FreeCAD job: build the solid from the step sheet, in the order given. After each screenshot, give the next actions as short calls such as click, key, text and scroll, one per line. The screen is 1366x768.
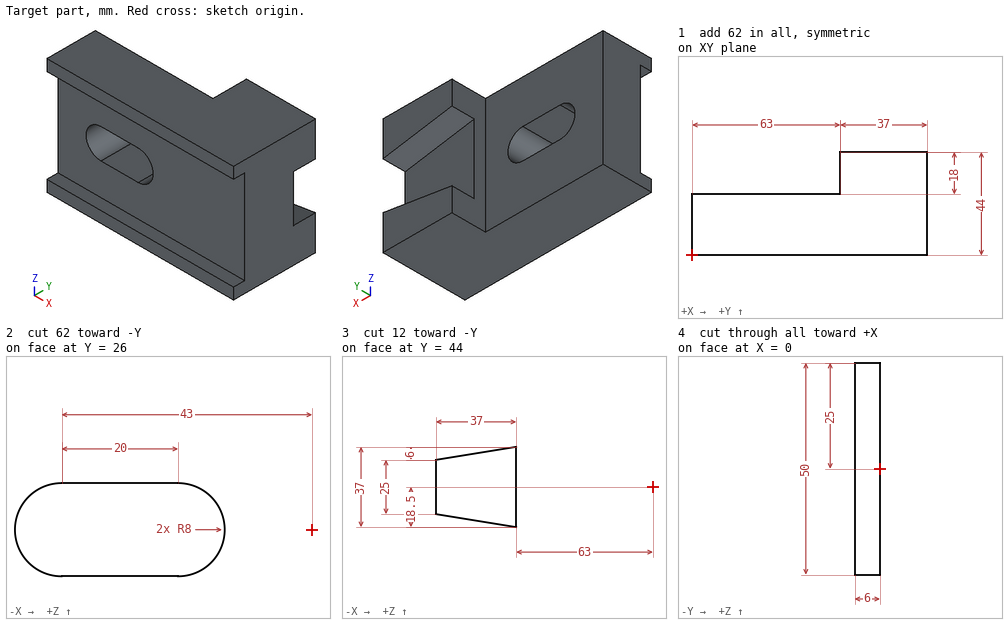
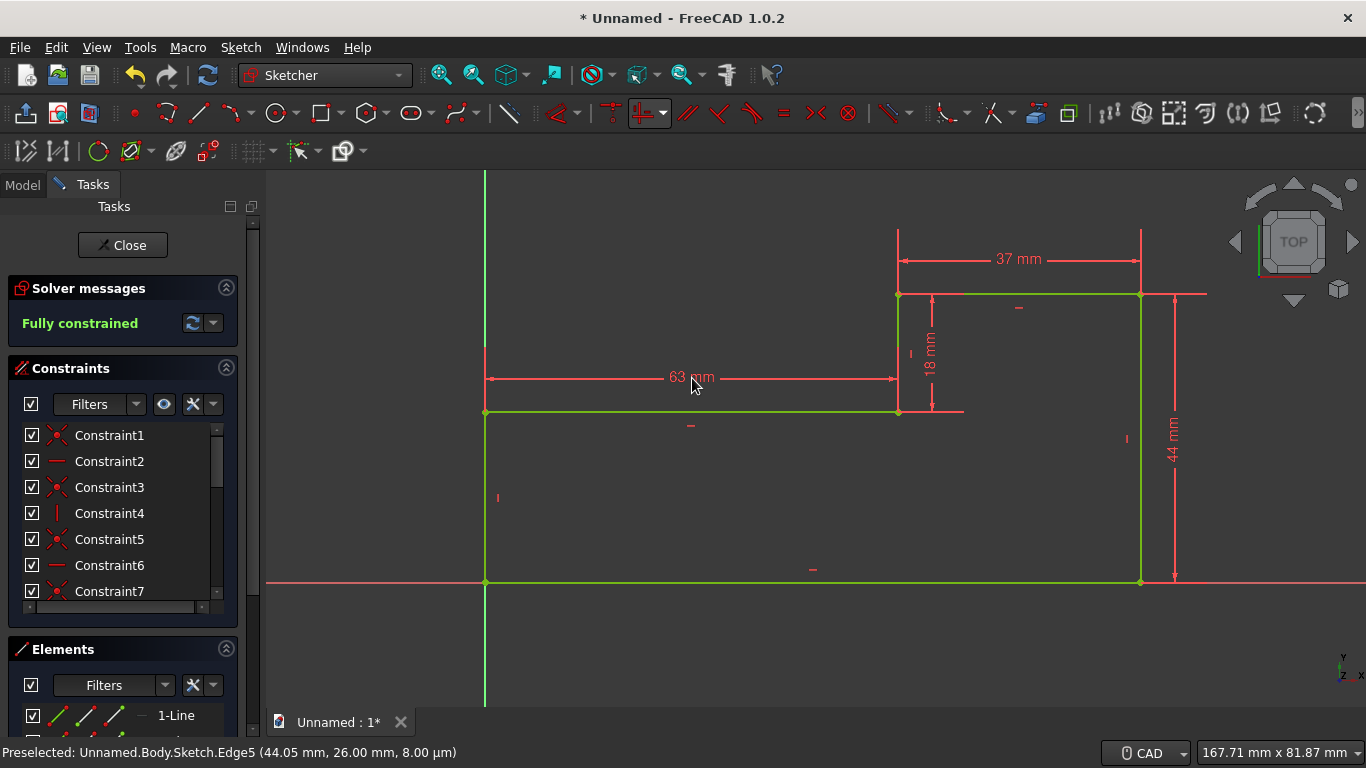
click(123, 245)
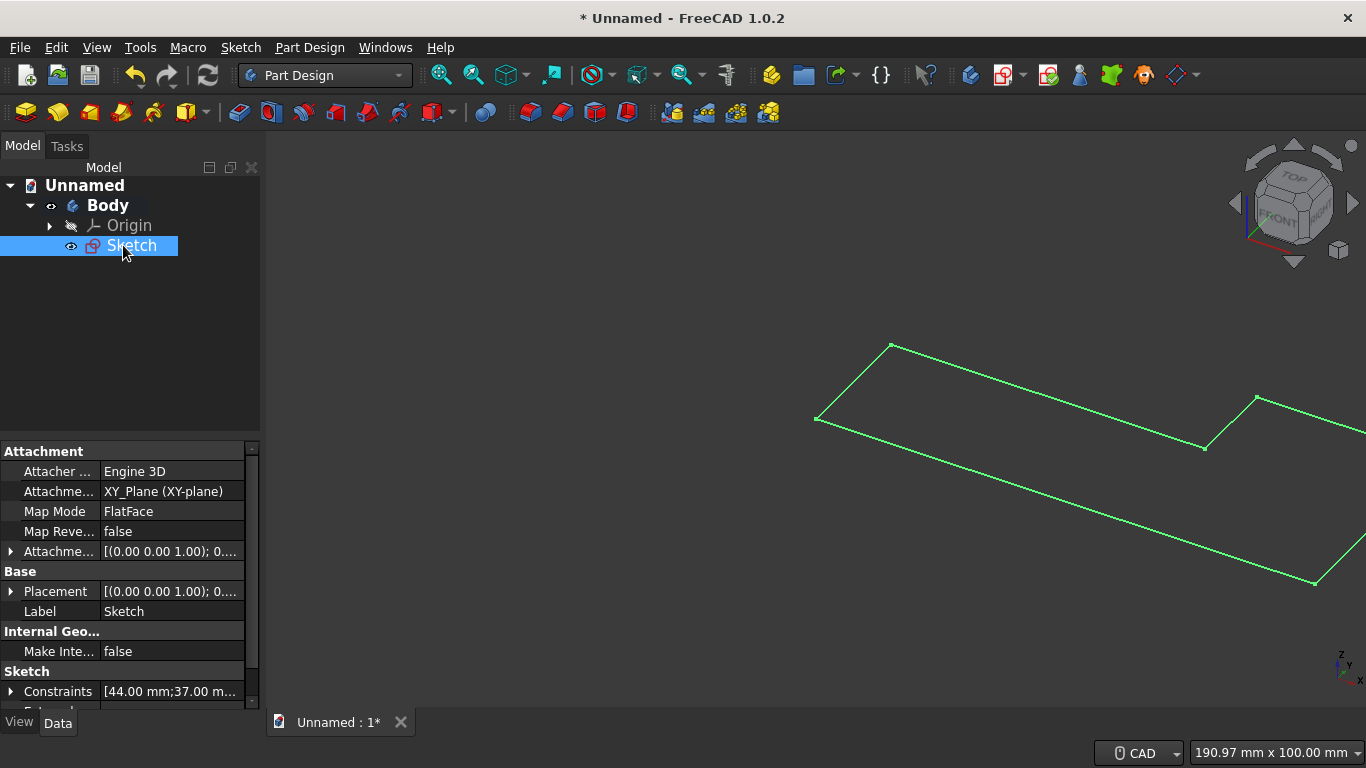
click(26, 112)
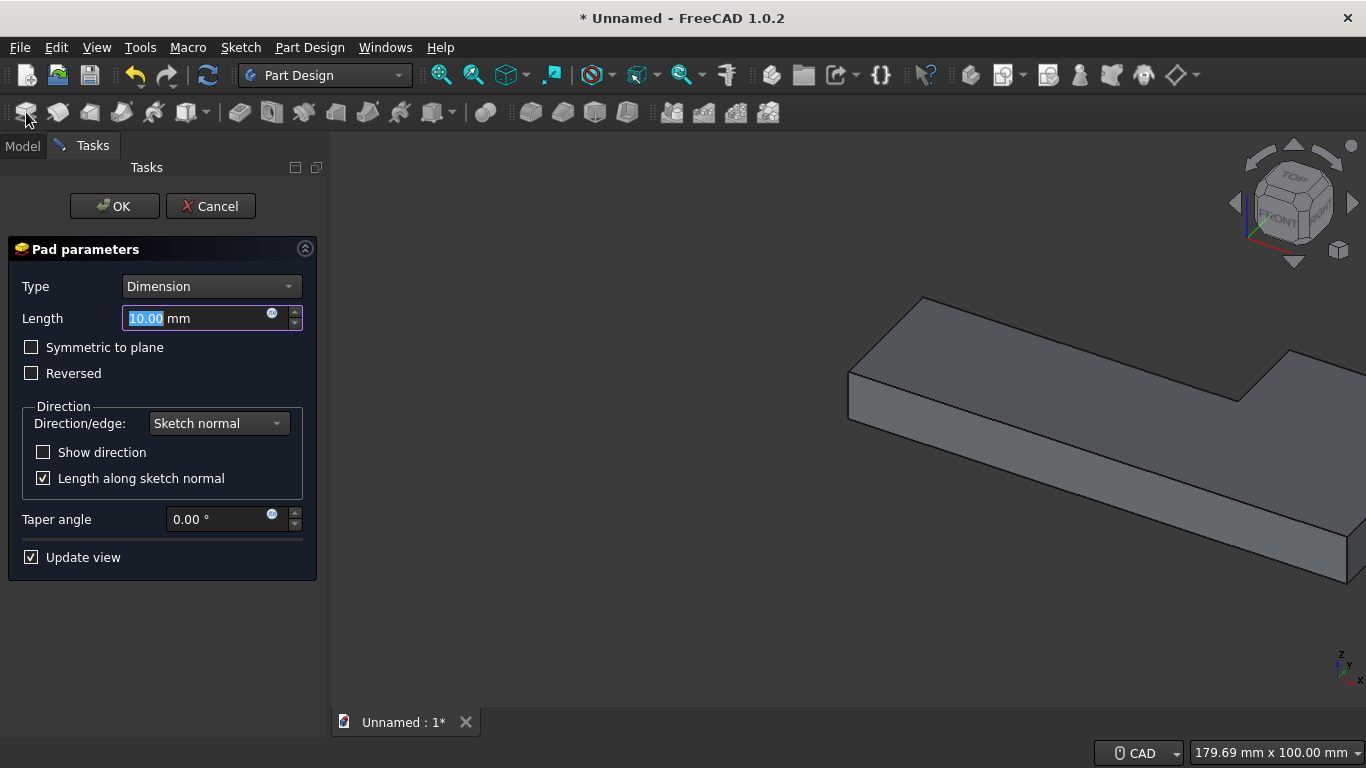
text(62)
key(Tab)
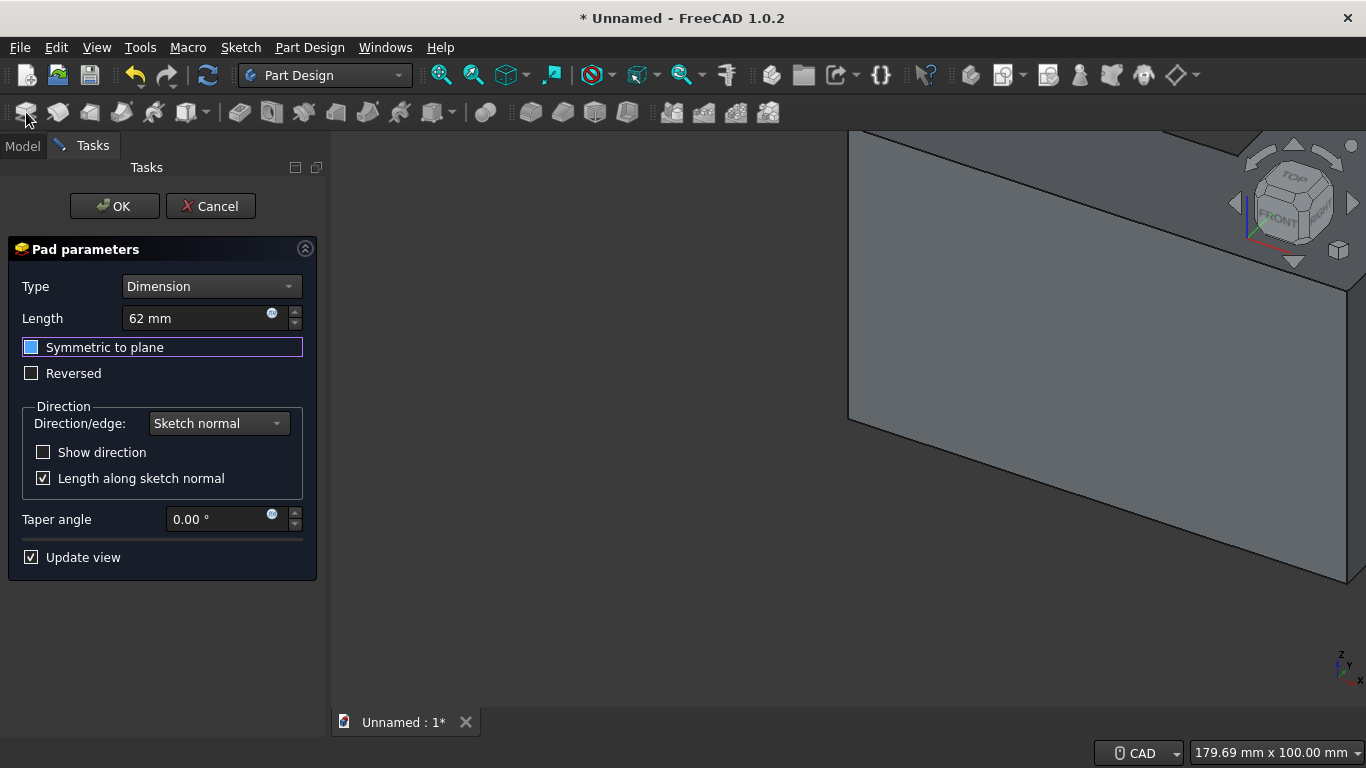
click(30, 347)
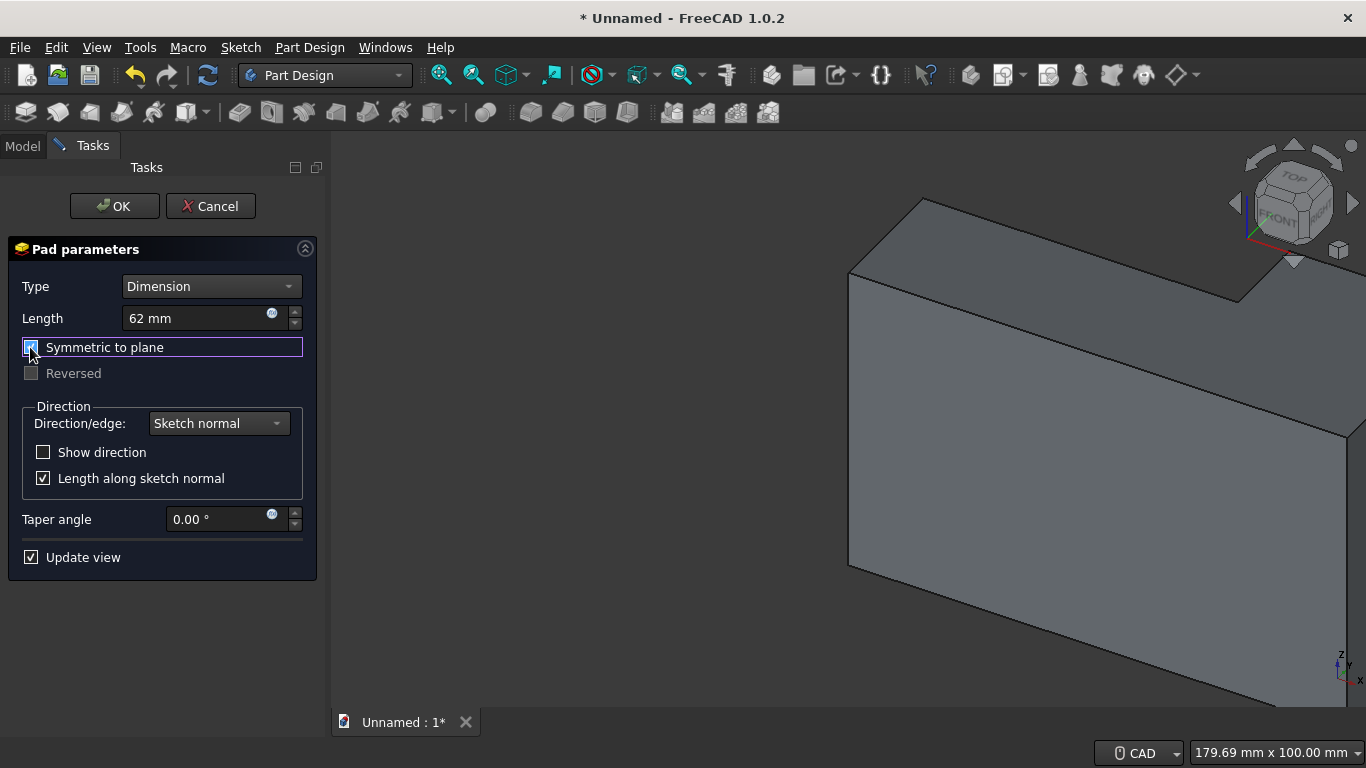
click(115, 206)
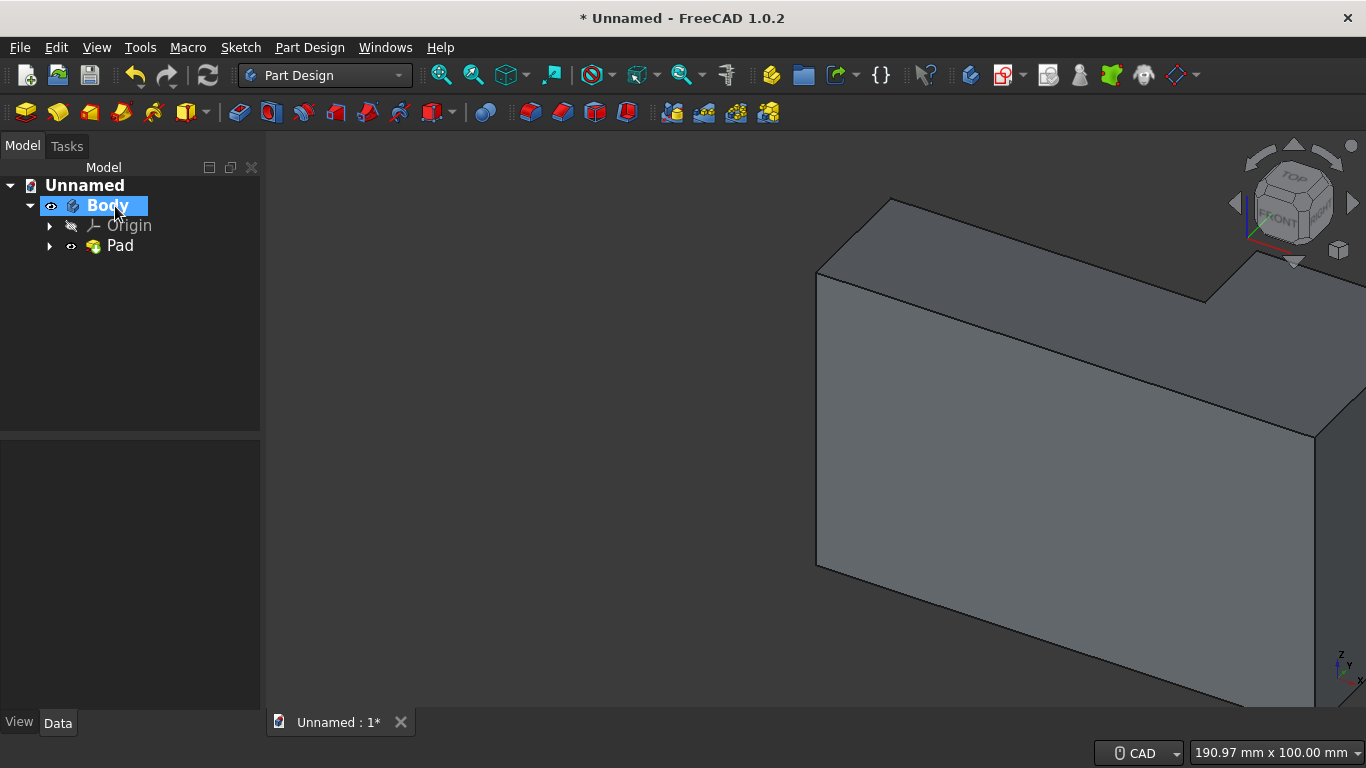
click(442, 76)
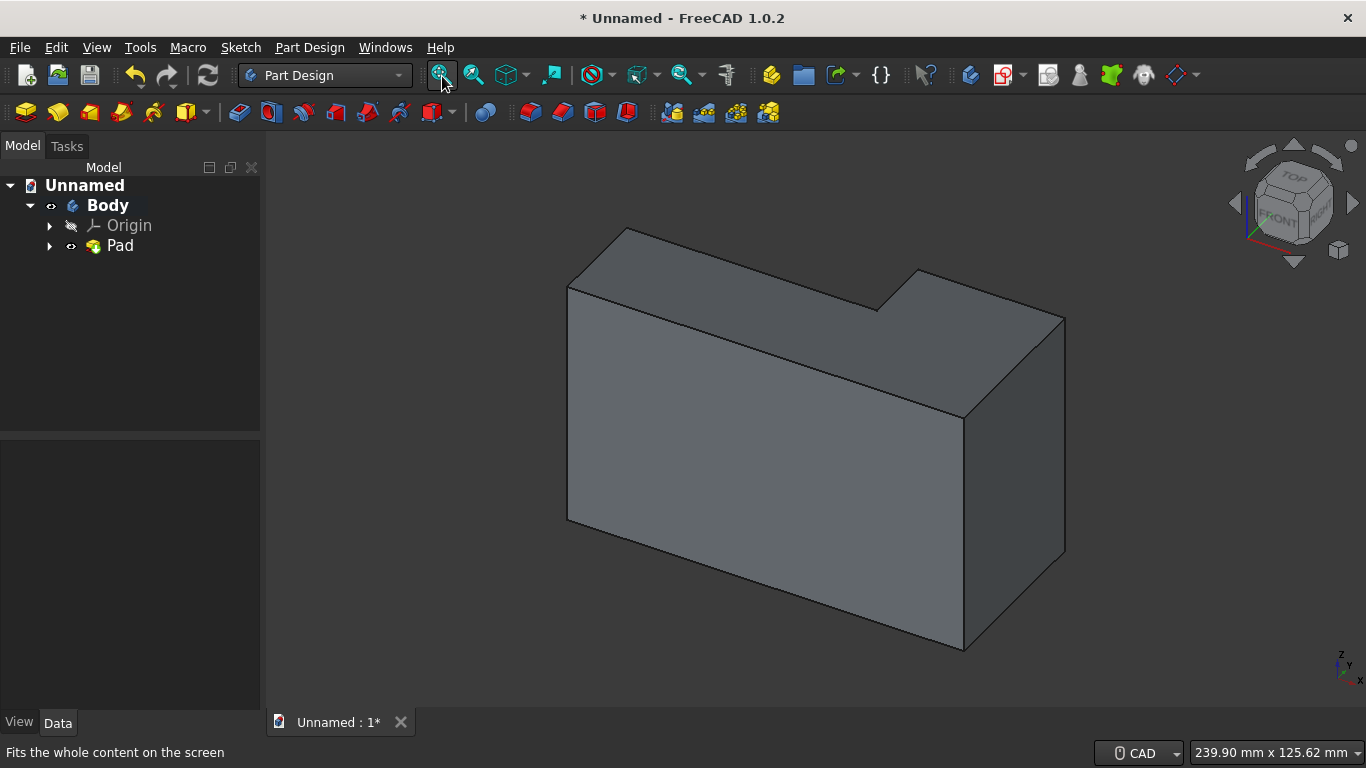
key(4)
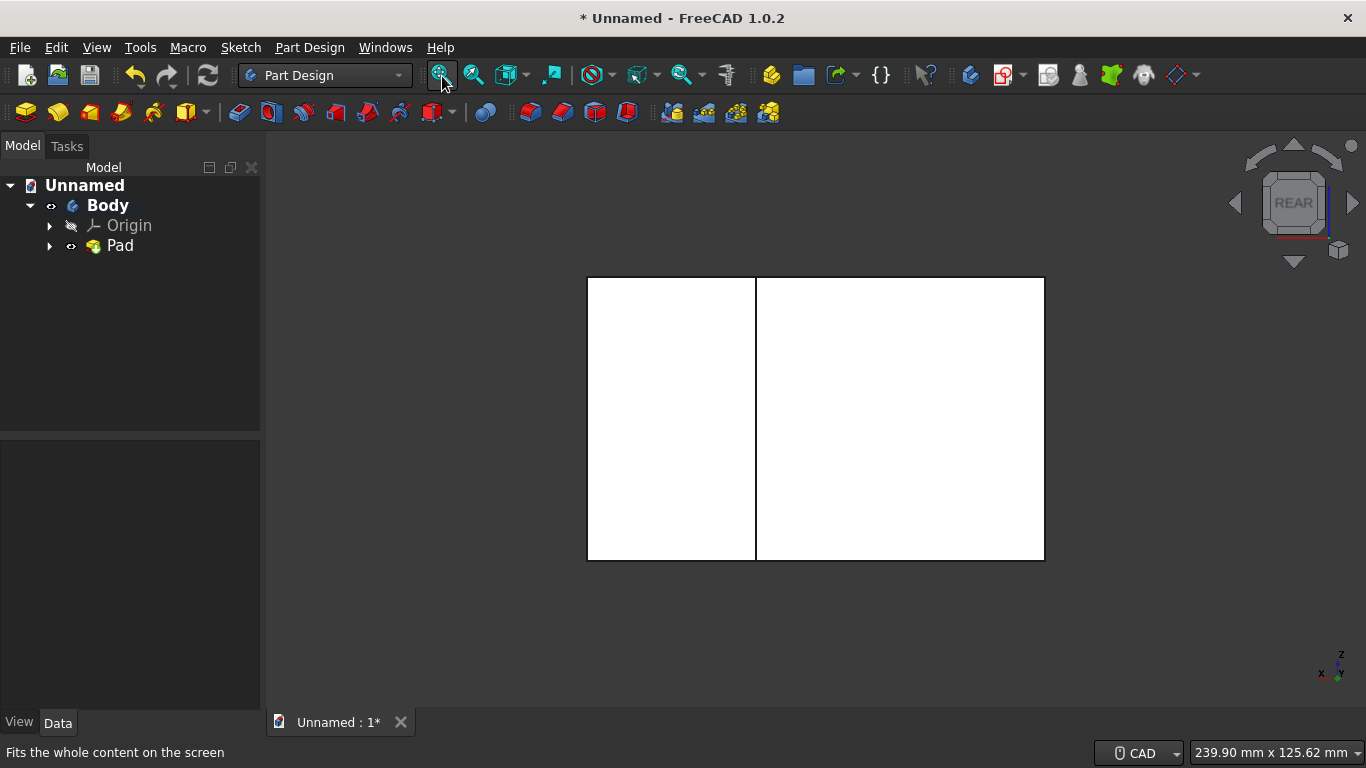
click(901, 418)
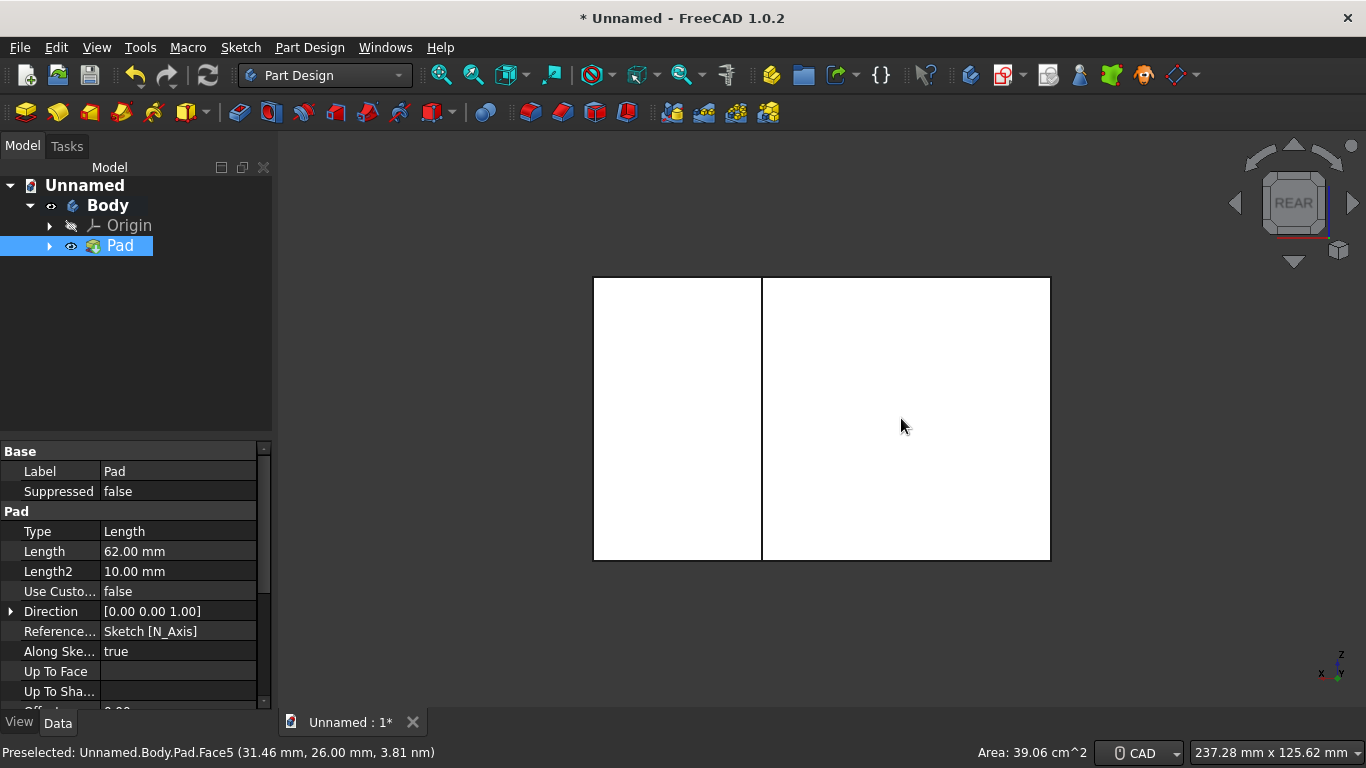
click(1004, 76)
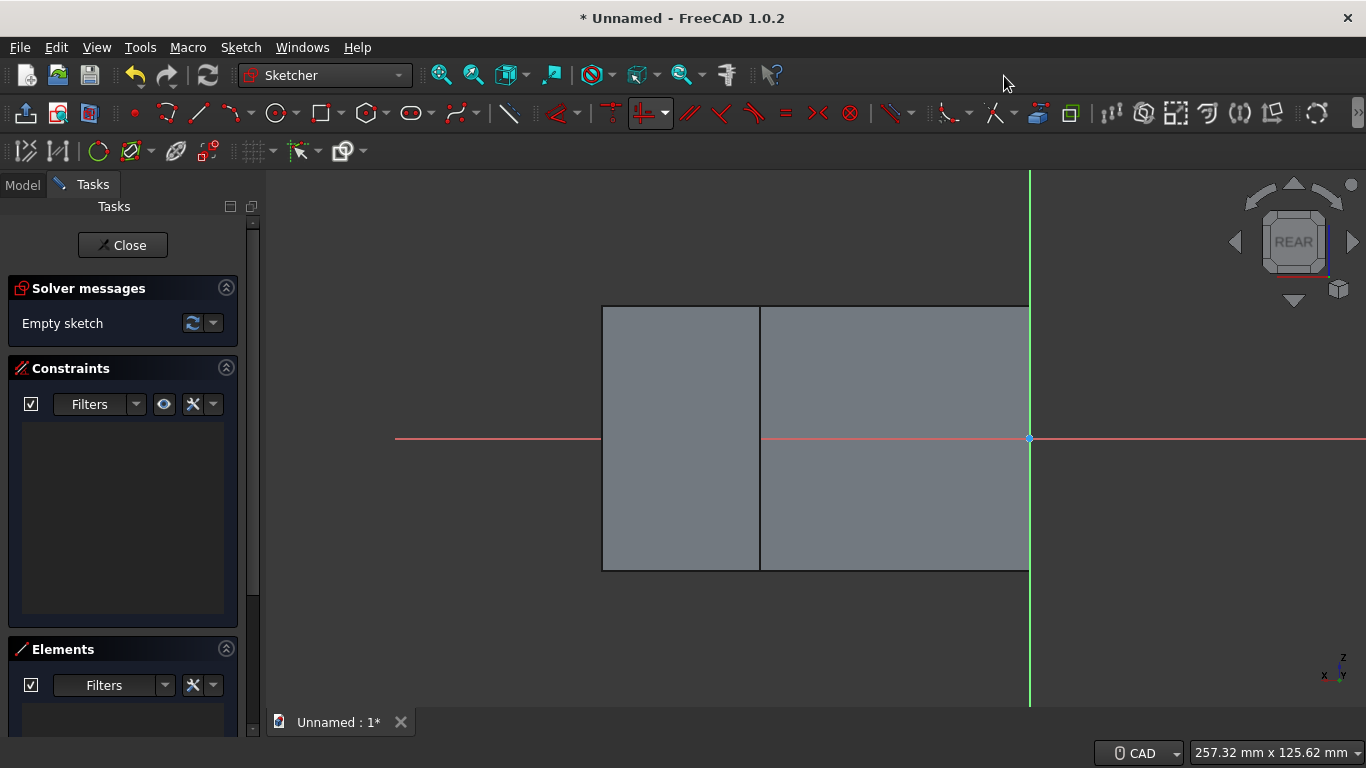
scroll(1022, 439, up, 5)